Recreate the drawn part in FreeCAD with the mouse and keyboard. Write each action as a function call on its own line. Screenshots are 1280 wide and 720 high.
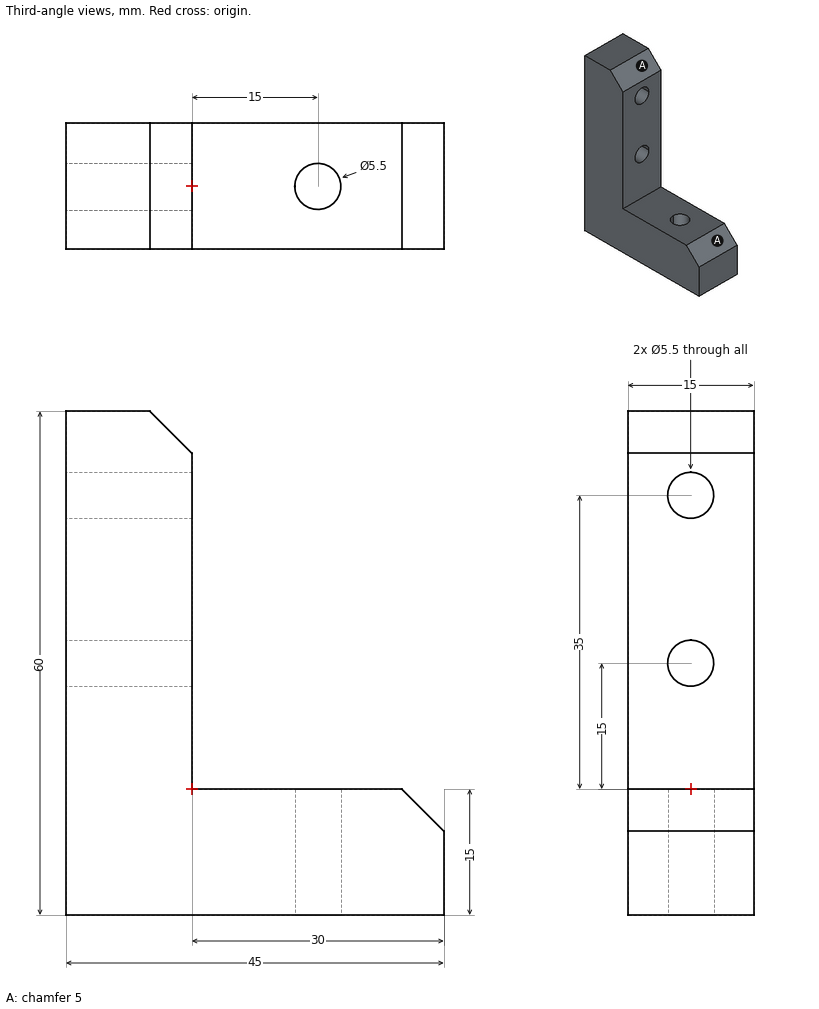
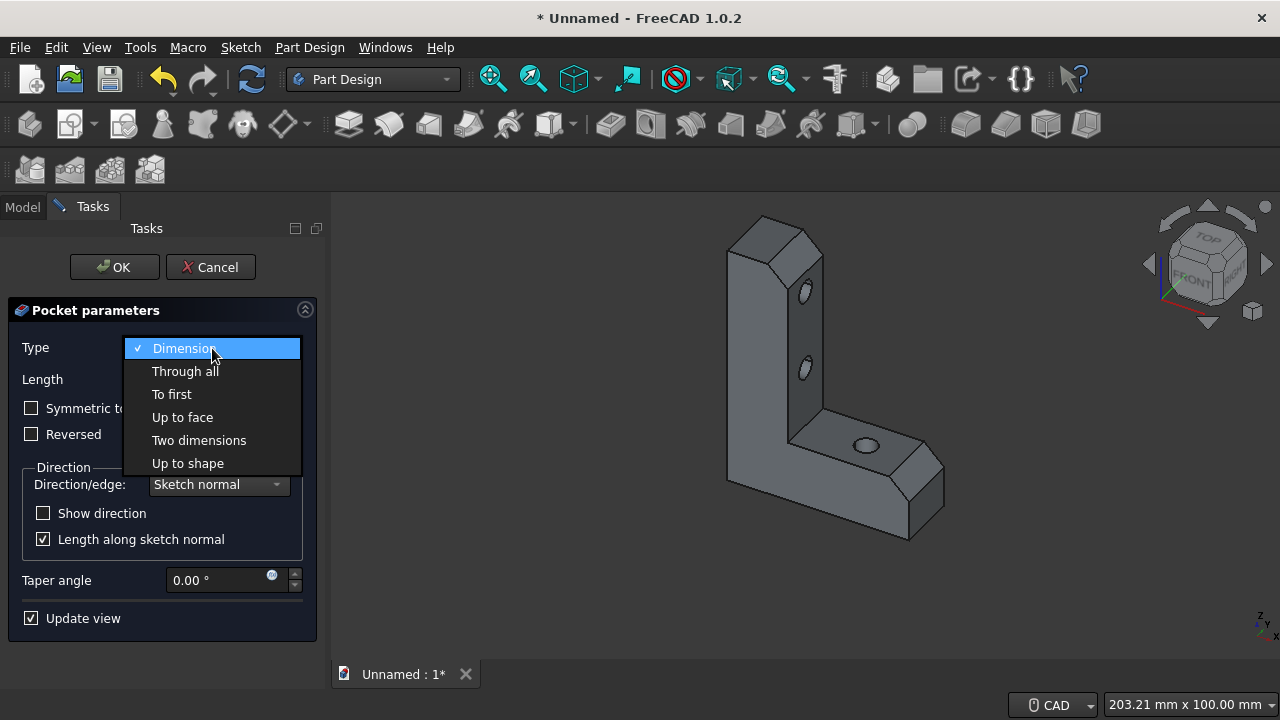
click(212, 372)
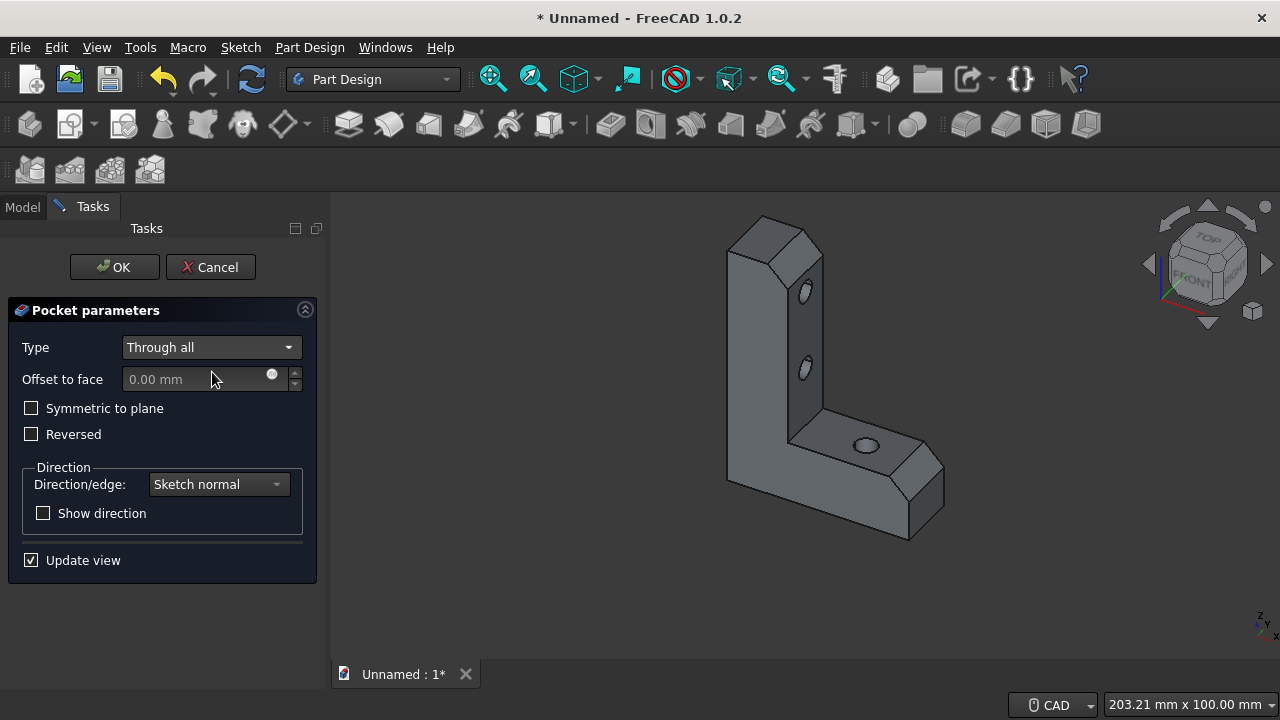
click(115, 267)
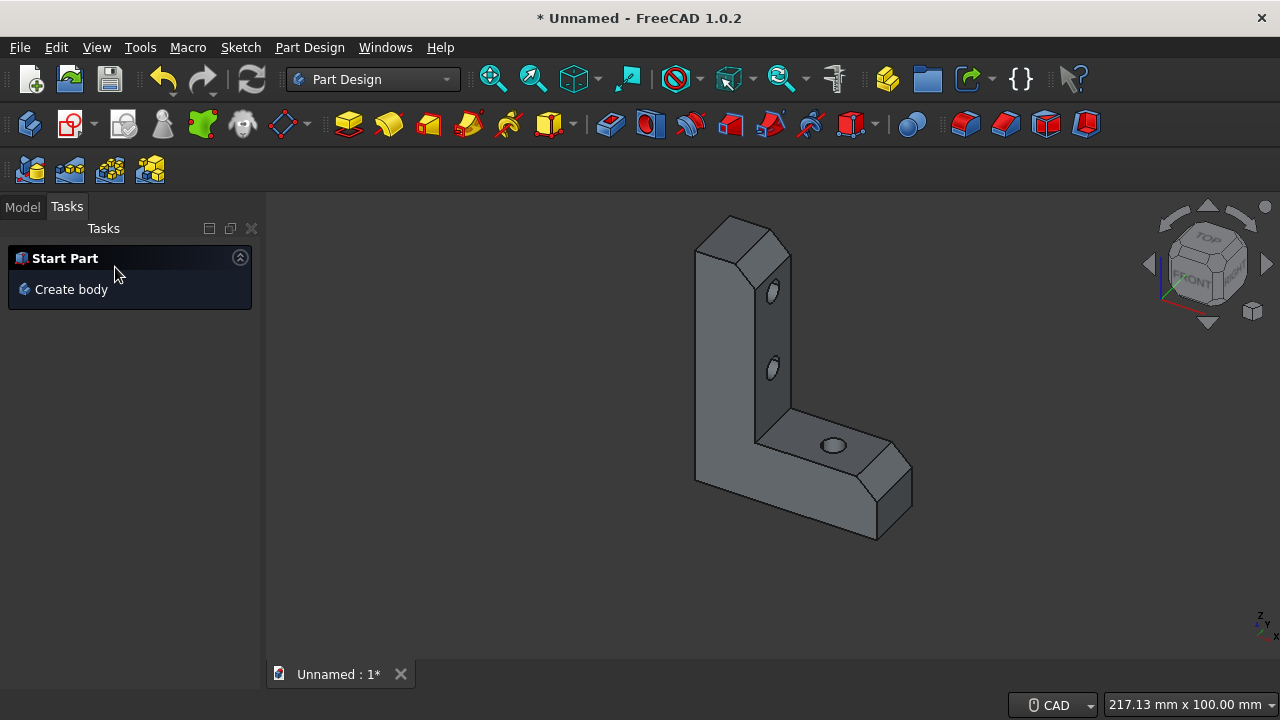
key(0)